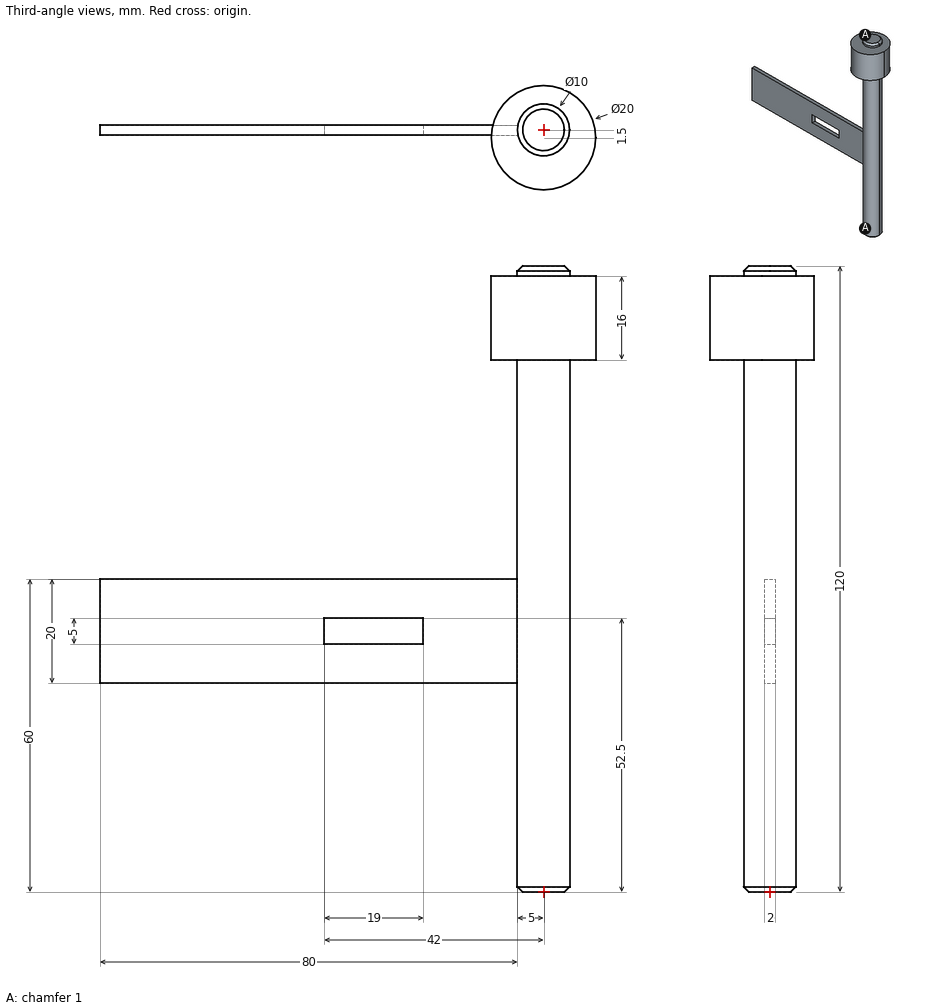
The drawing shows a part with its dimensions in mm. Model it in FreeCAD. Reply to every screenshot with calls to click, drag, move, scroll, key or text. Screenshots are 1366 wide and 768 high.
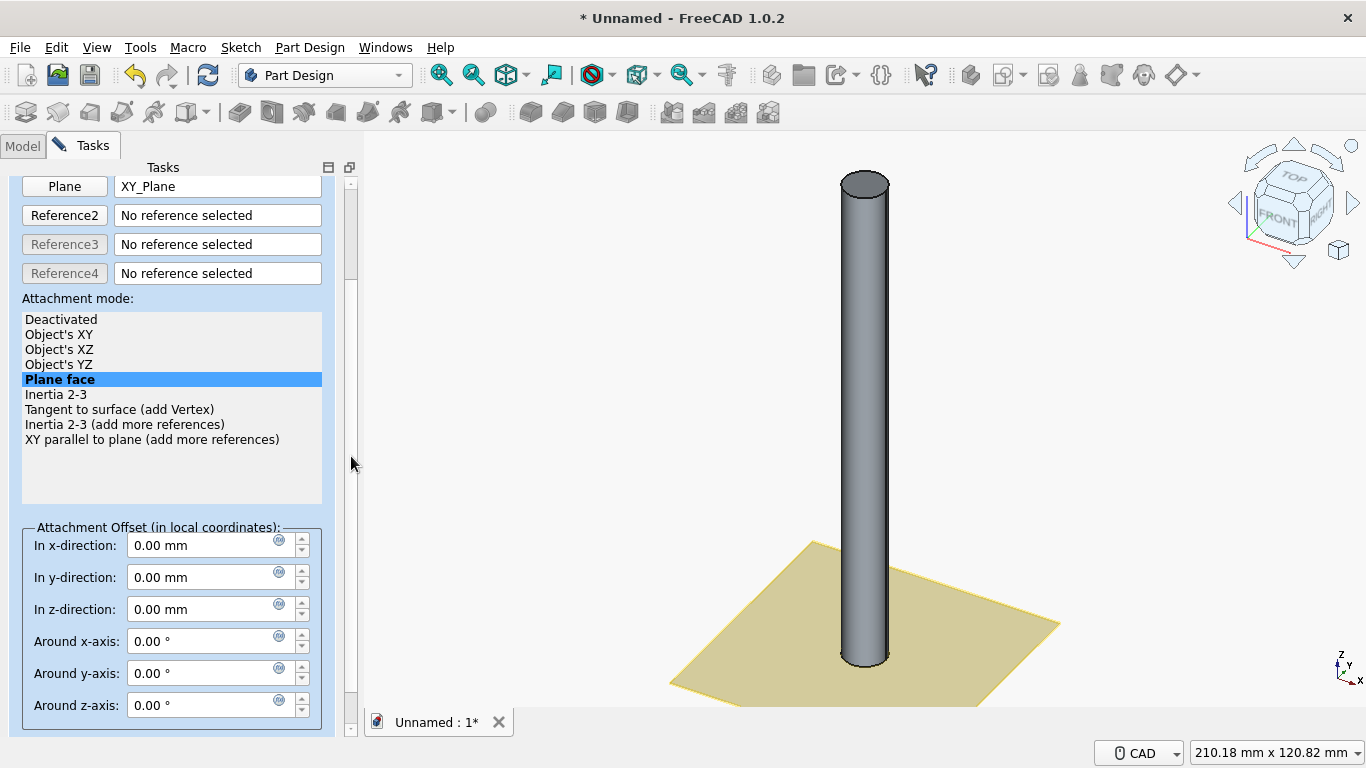
triple_click(210, 609)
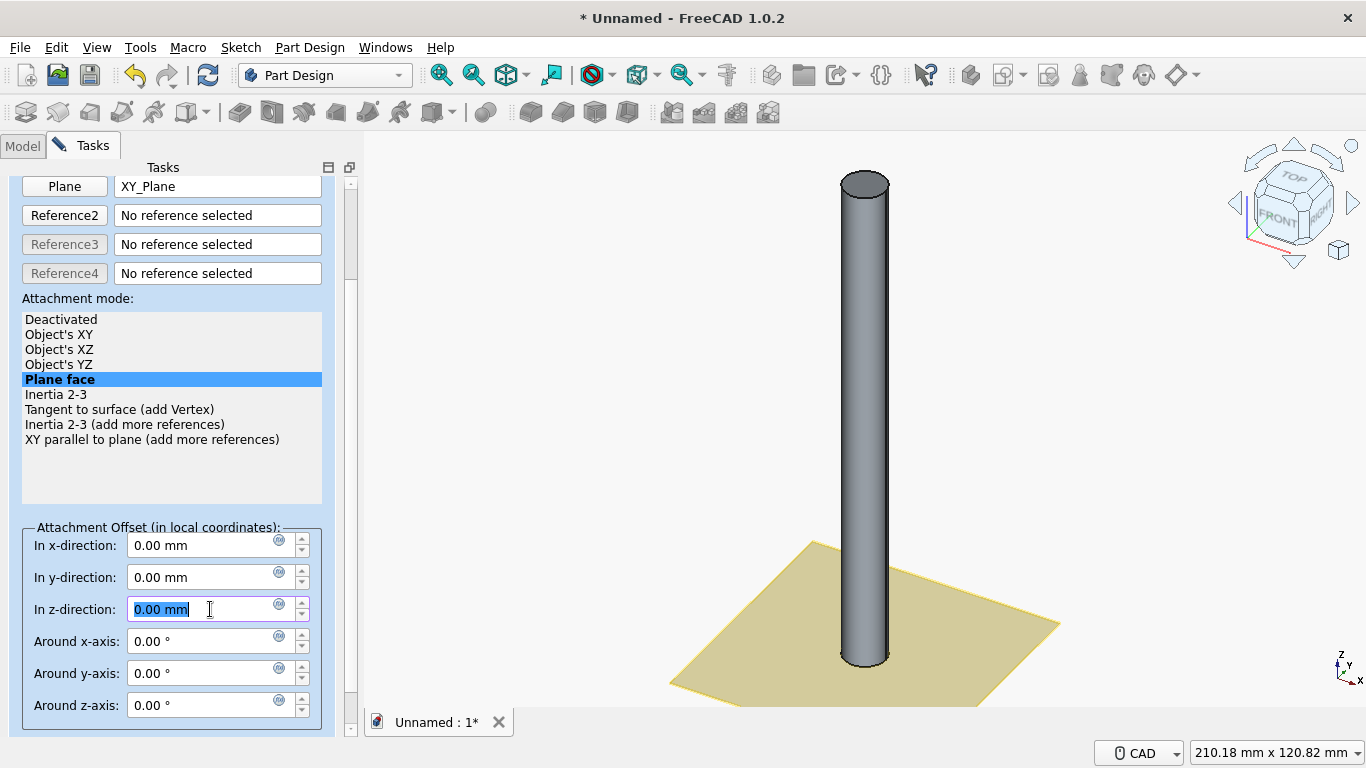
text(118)
key(Tab)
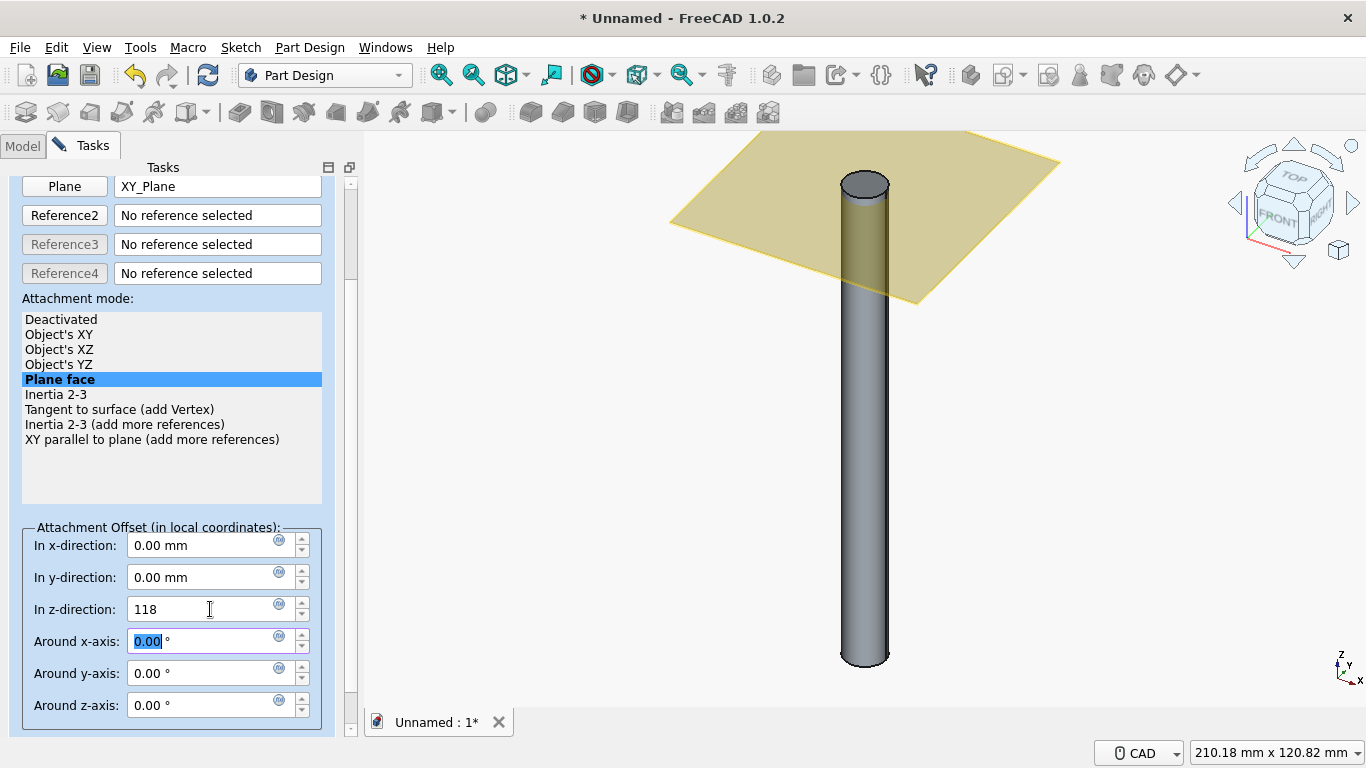
scroll(351, 456, up, 3)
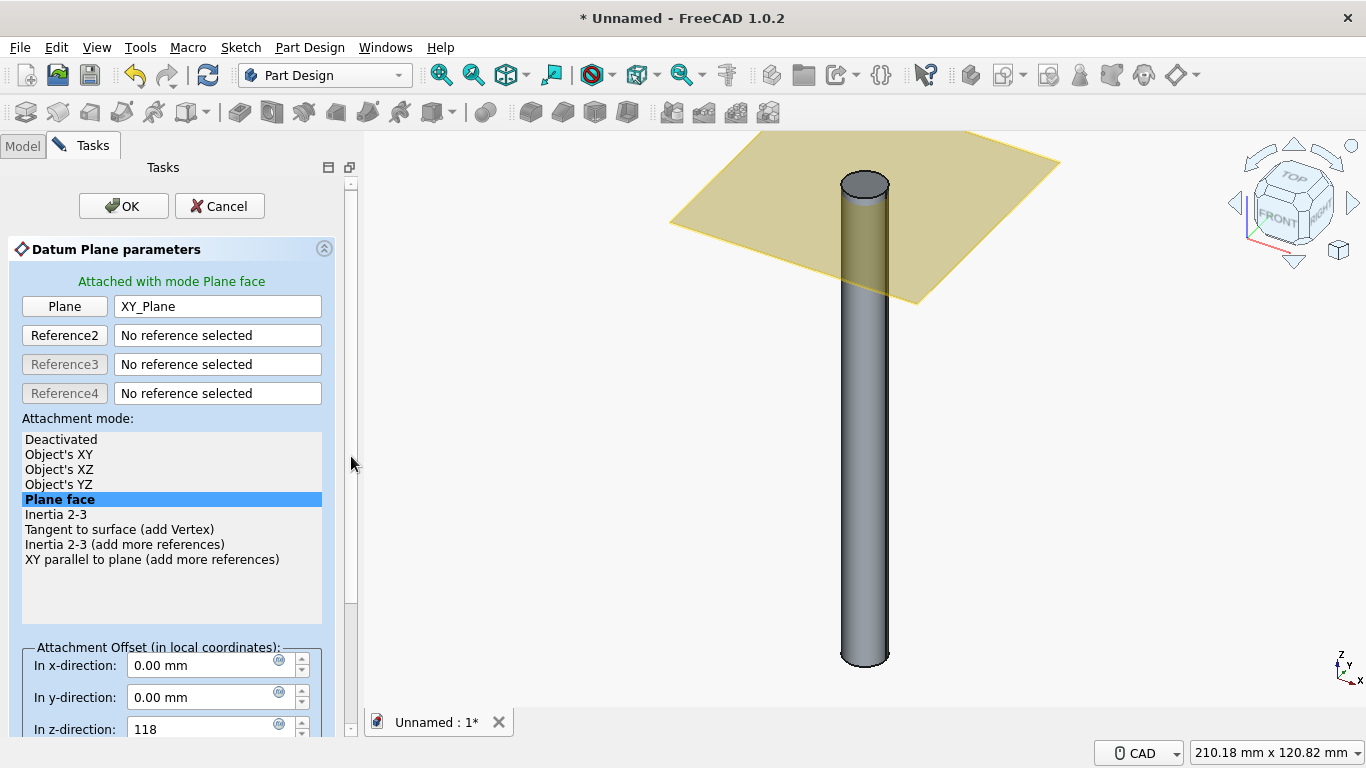
click(124, 206)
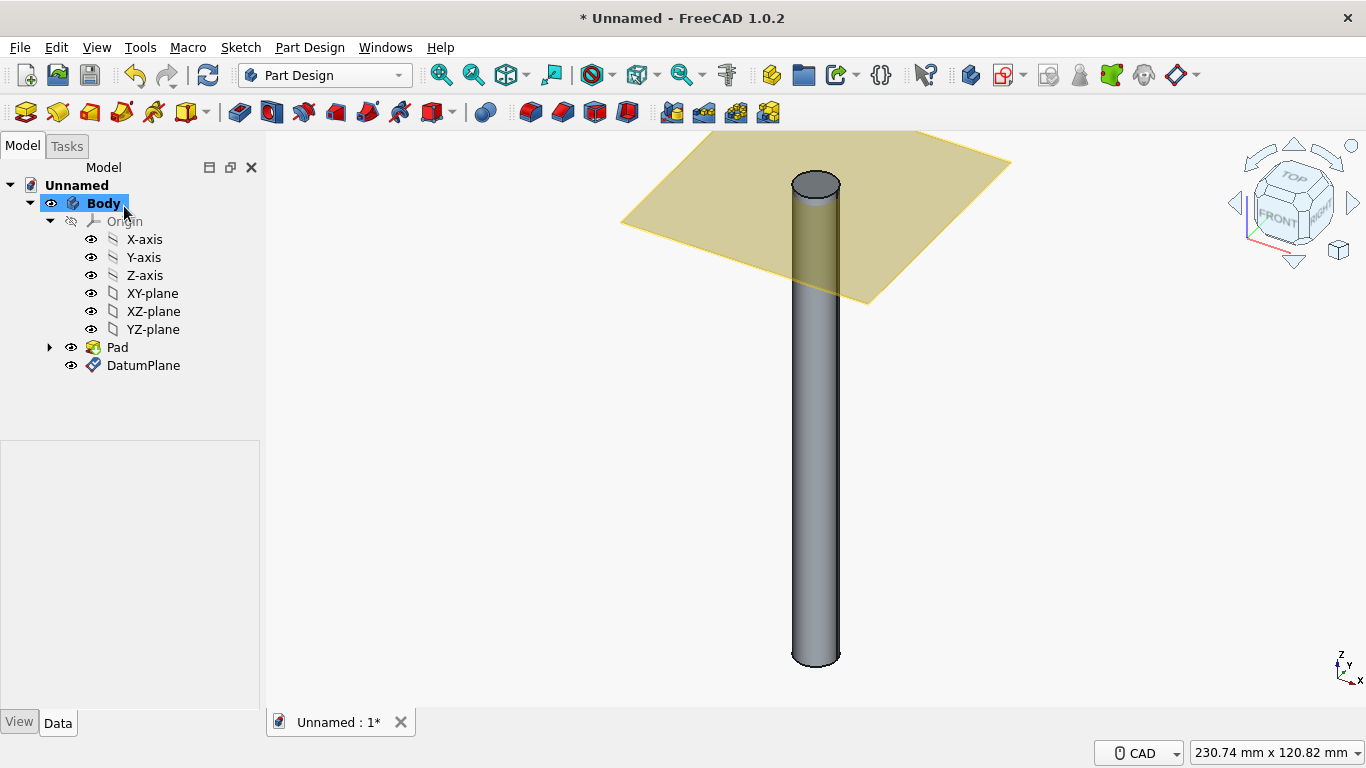
click(116, 365)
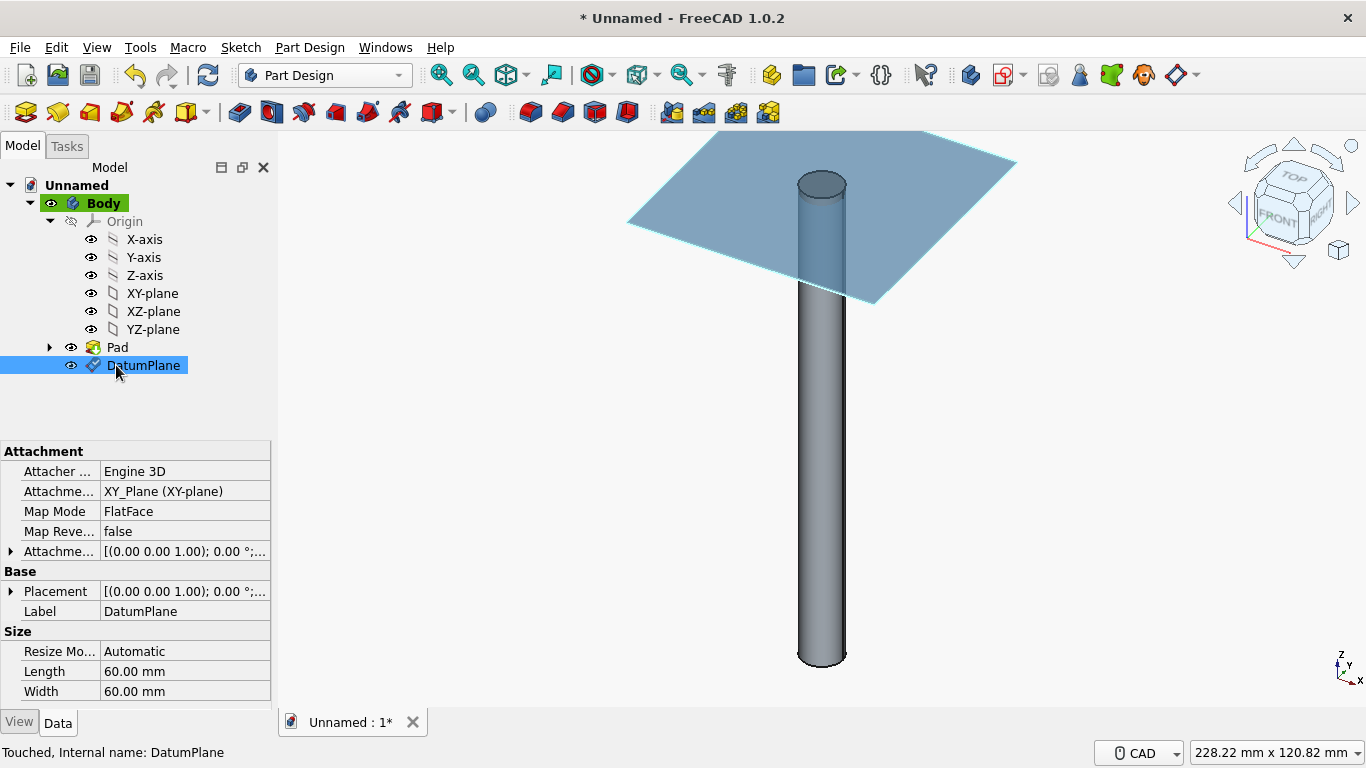
click(1004, 76)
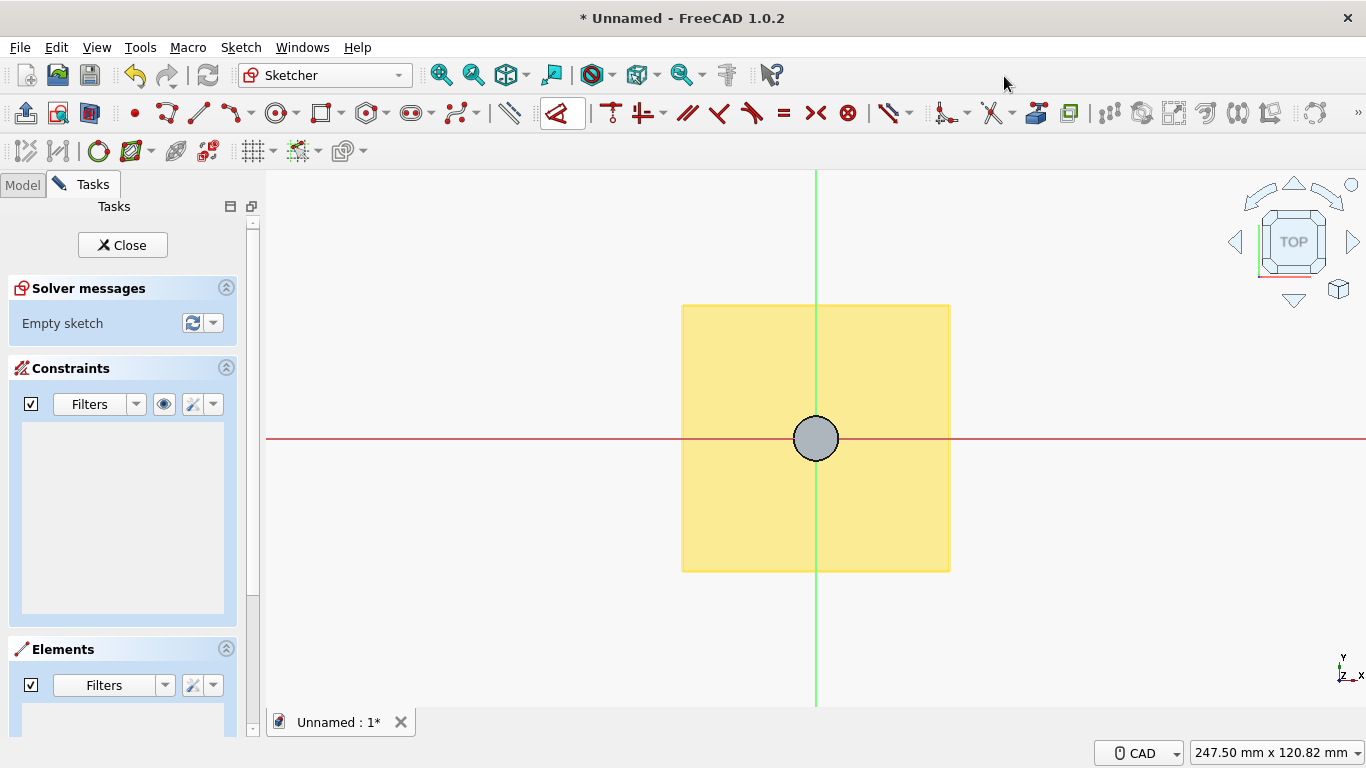
click(90, 114)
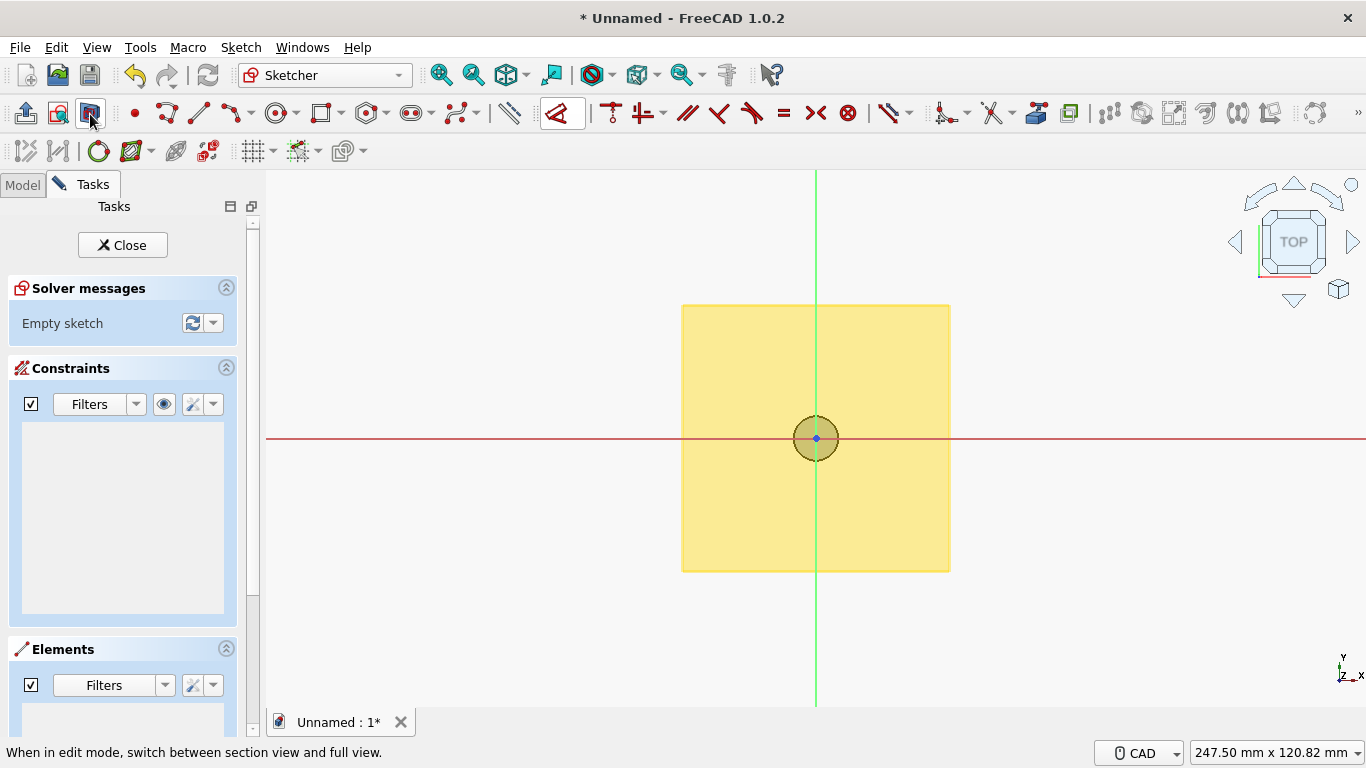
scroll(838, 447, up, 7)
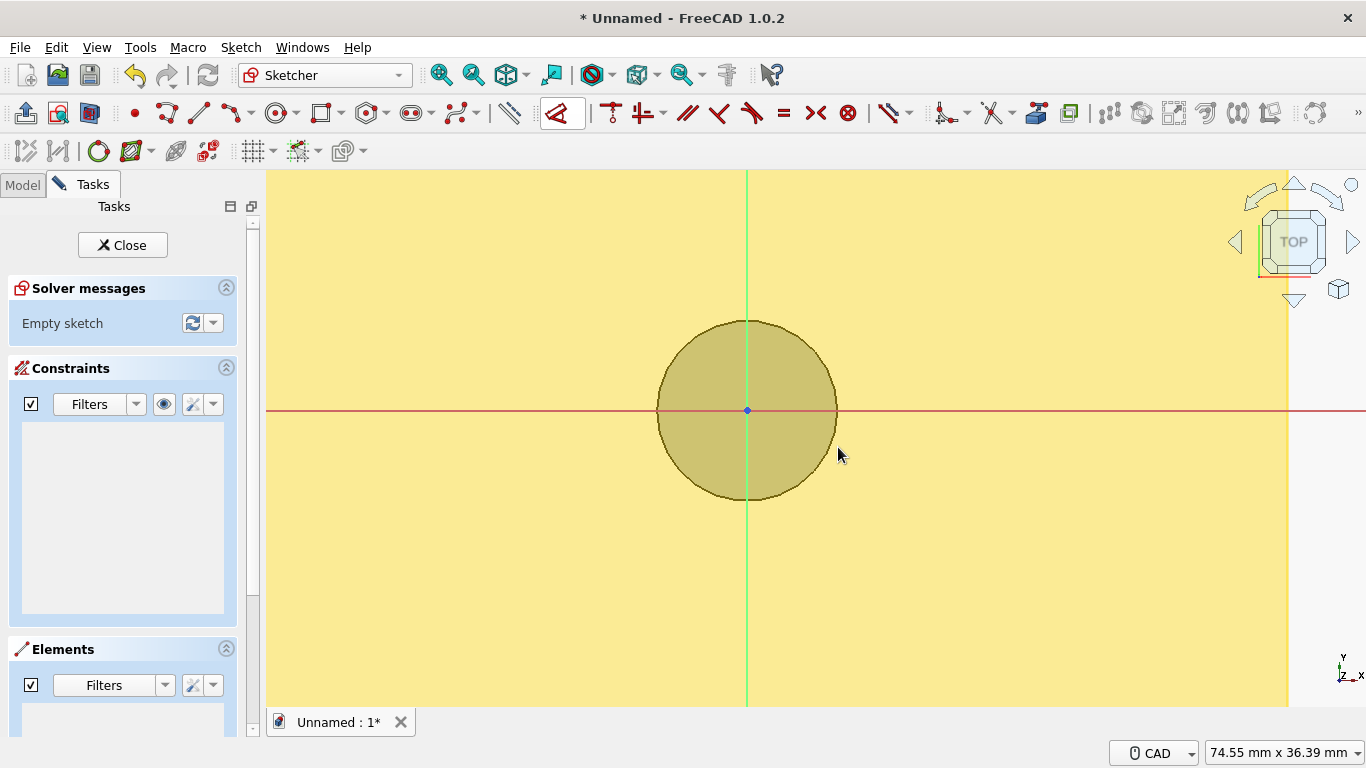
click(276, 114)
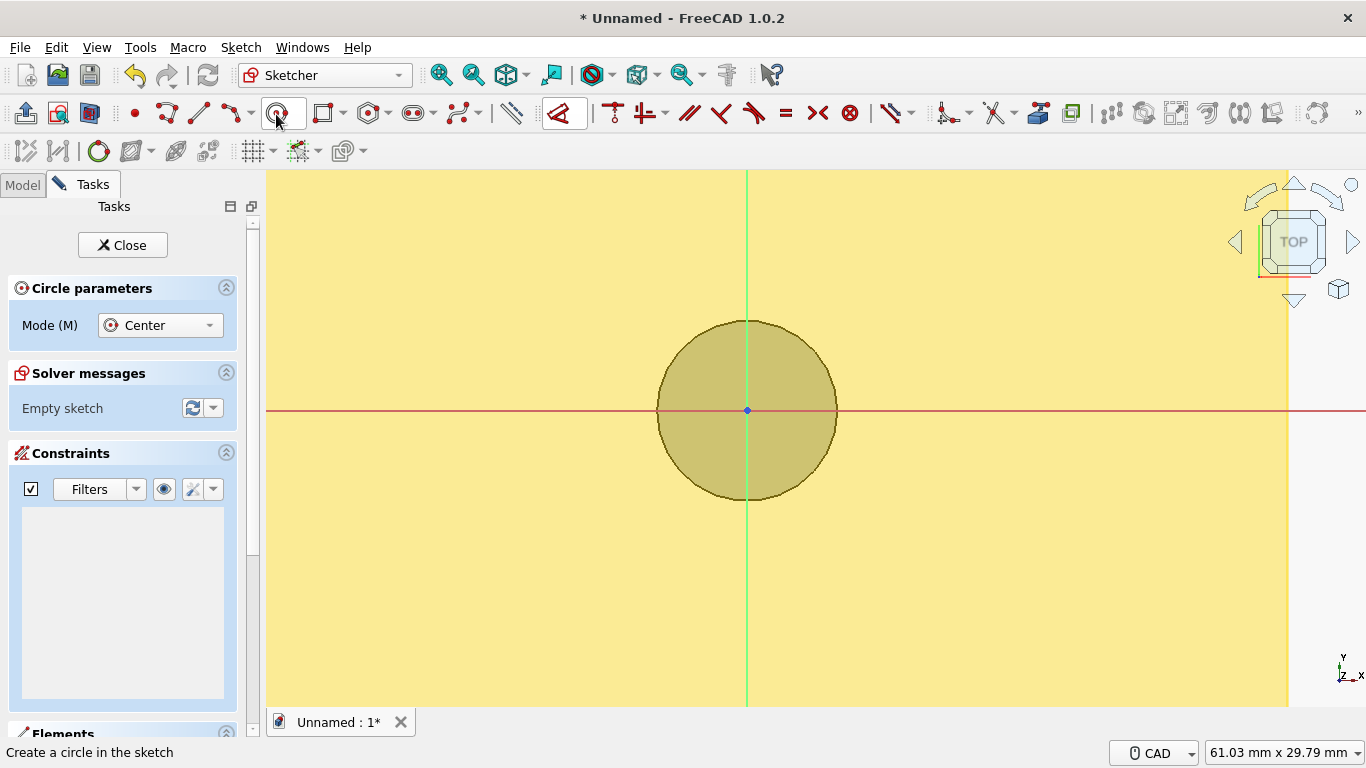
click(747, 438)
click(875, 311)
key(Escape)